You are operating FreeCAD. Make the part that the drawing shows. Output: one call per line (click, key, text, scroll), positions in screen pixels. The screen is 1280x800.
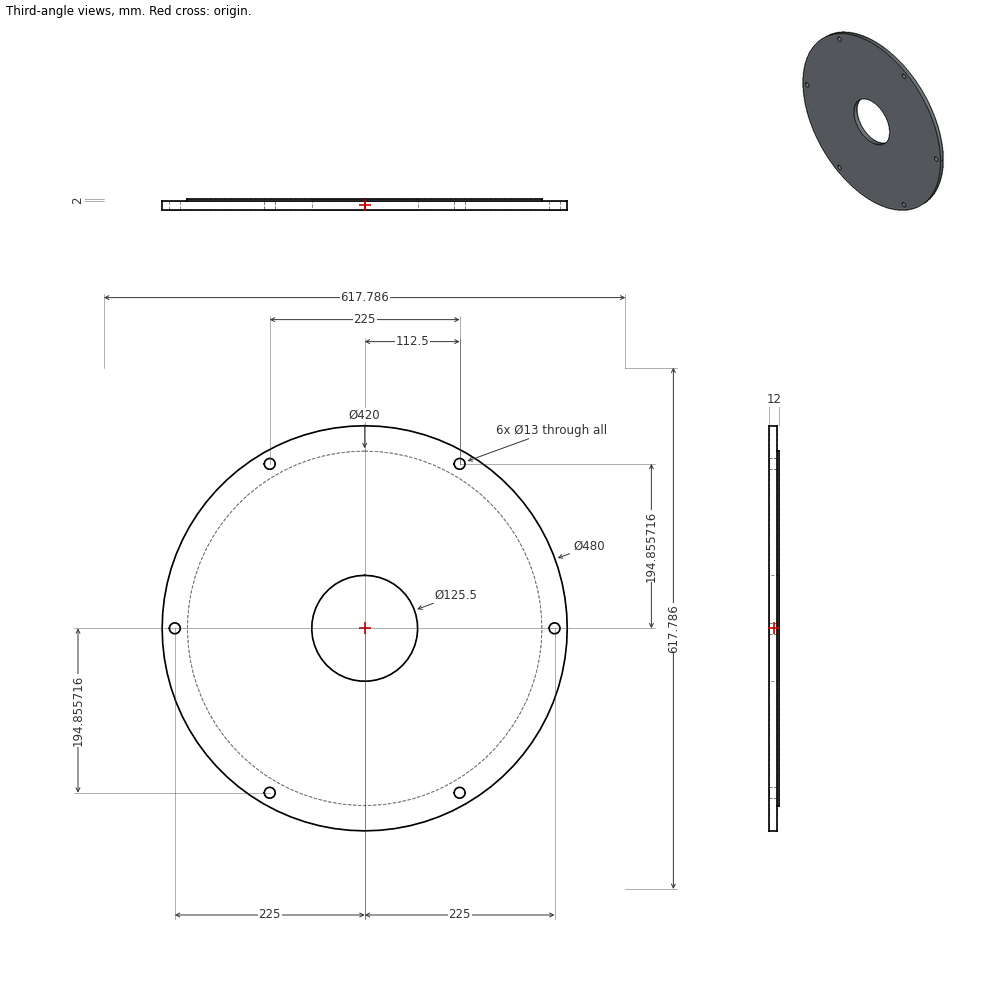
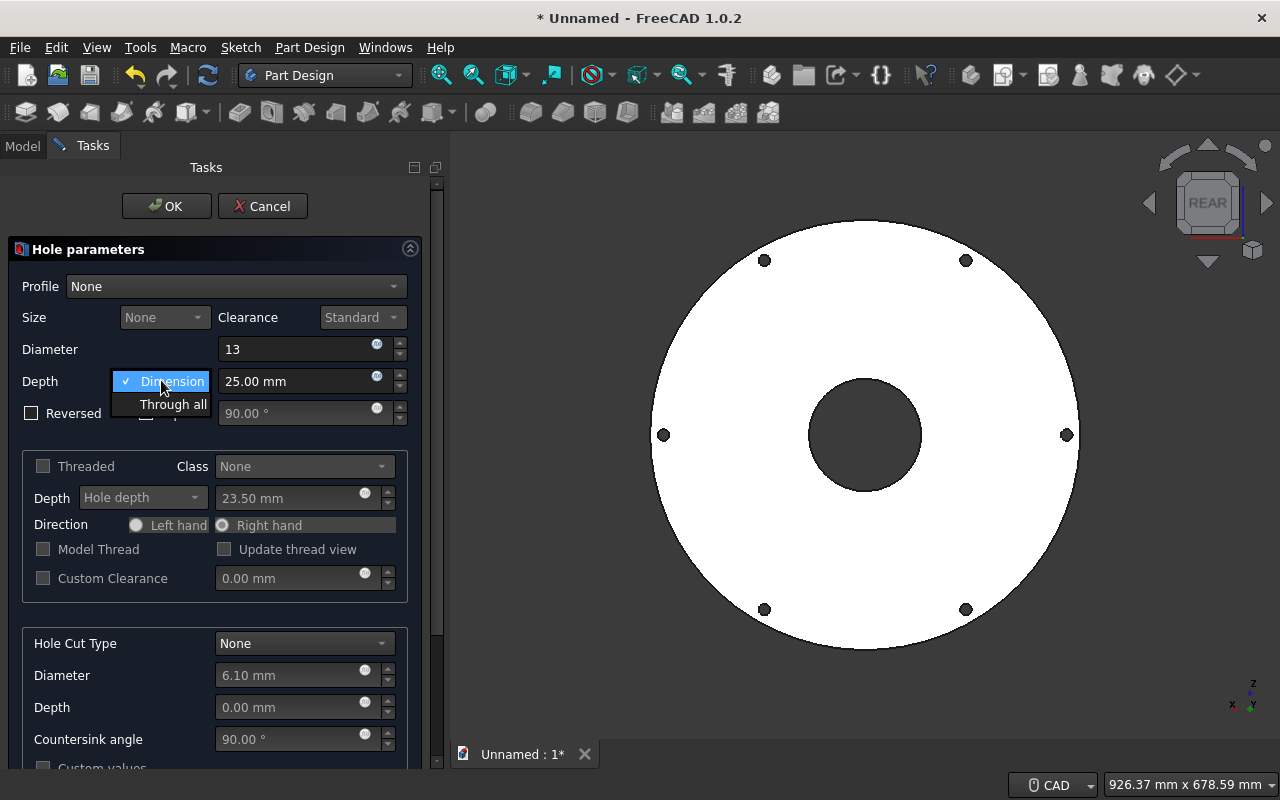
click(160, 404)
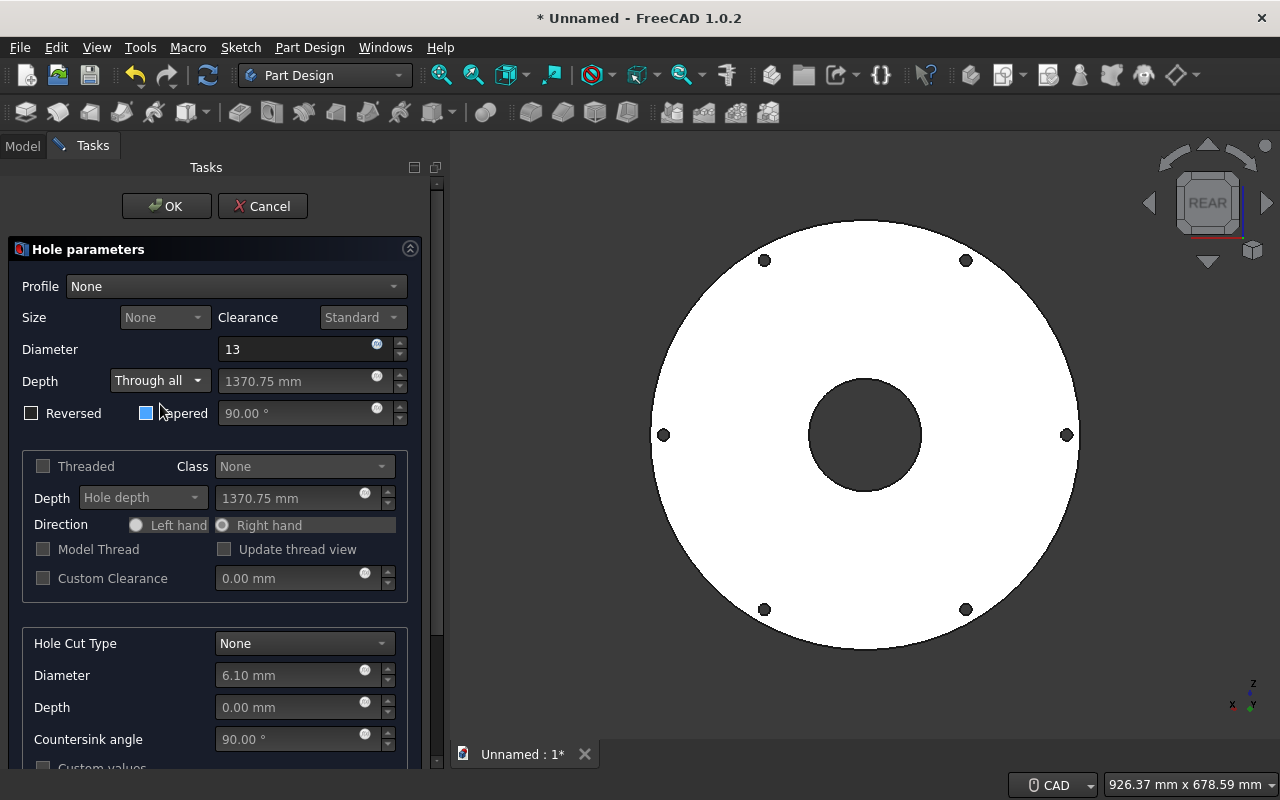
click(167, 206)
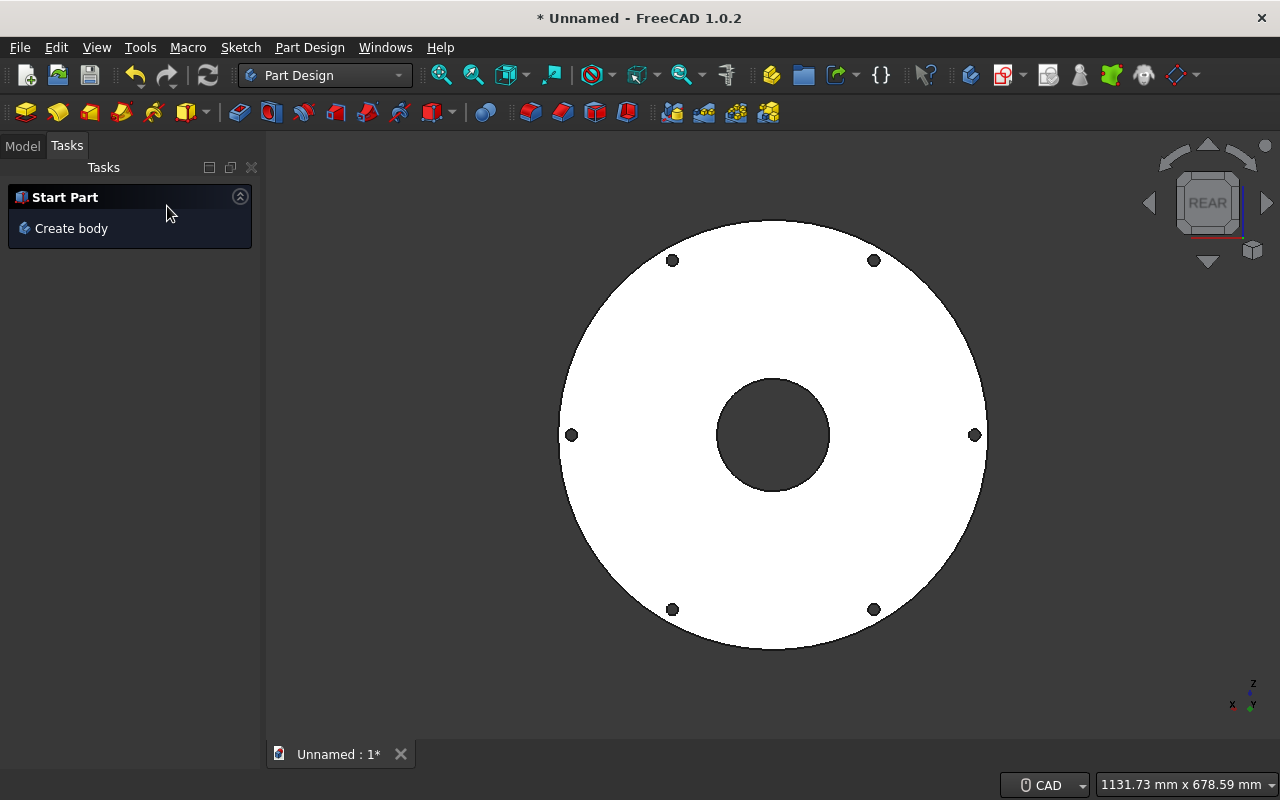
click(896, 373)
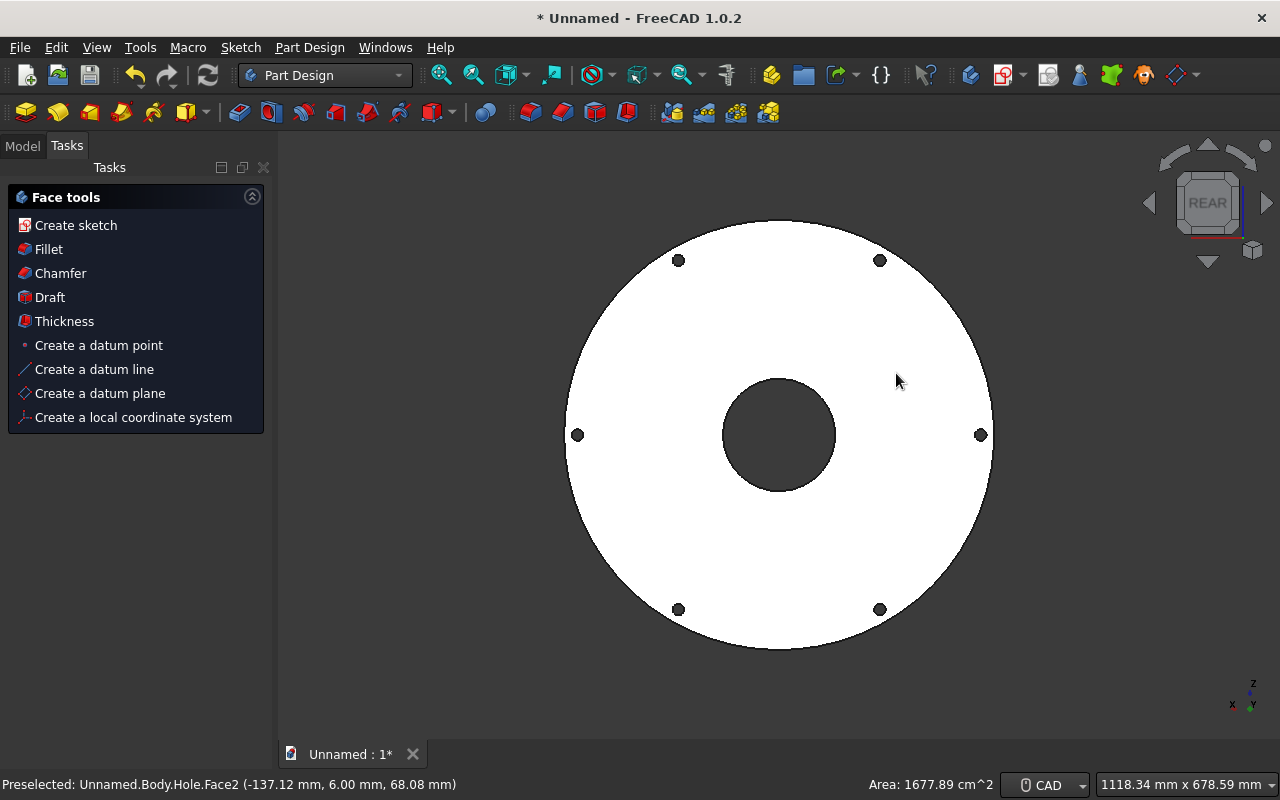
click(1004, 76)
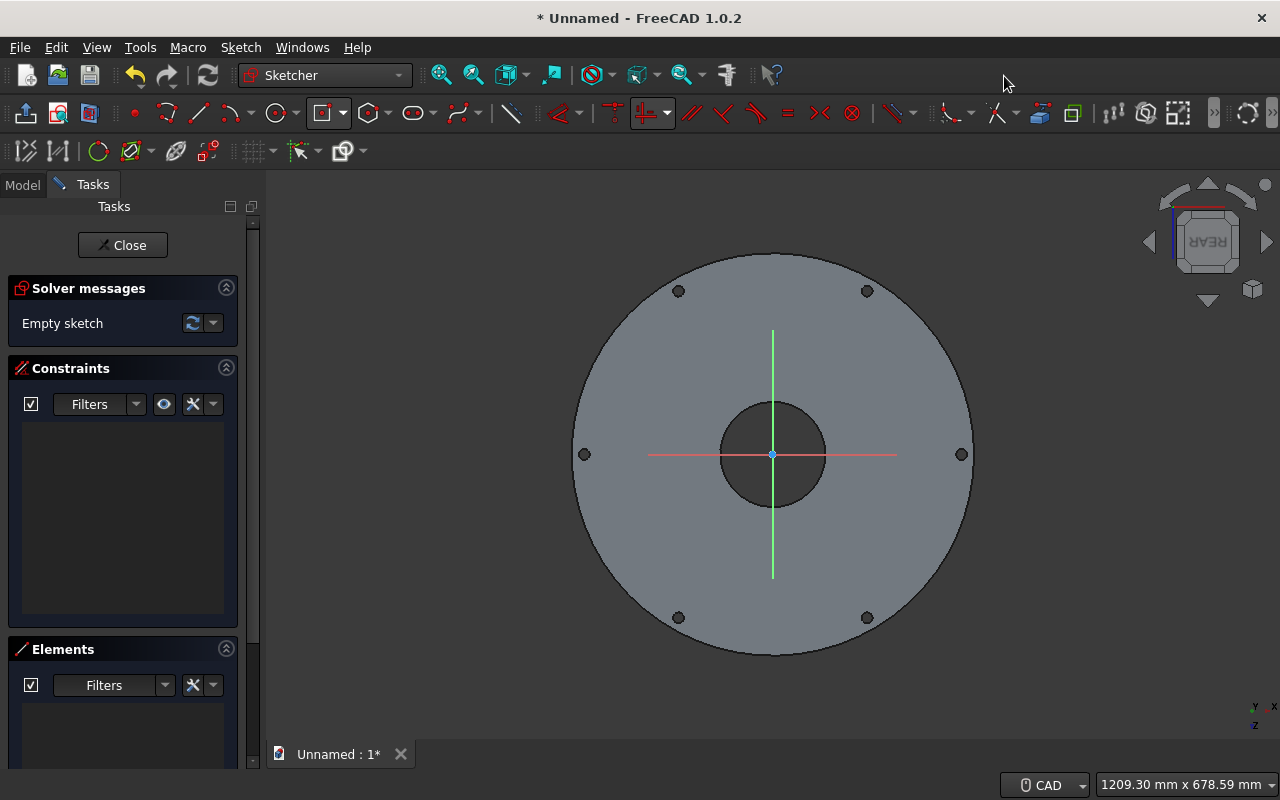
scroll(565, 455, down, 2)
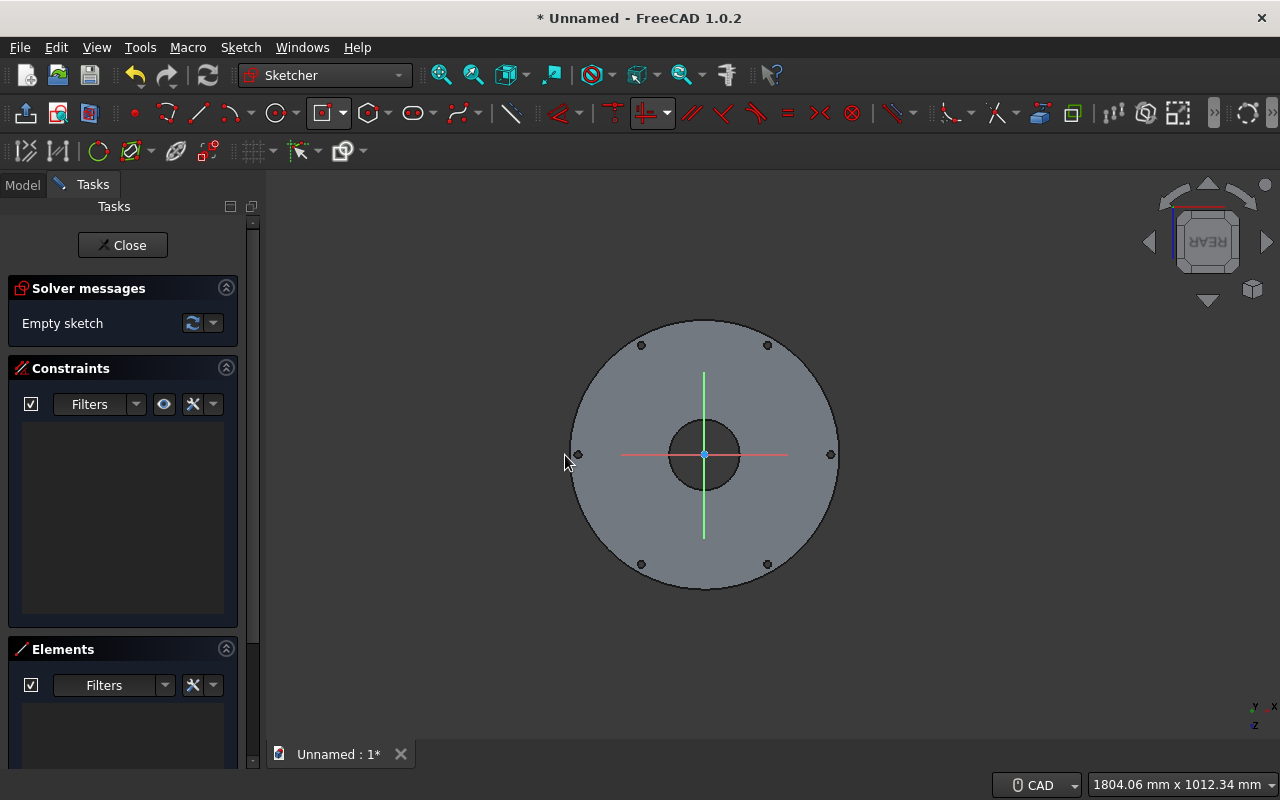
click(322, 114)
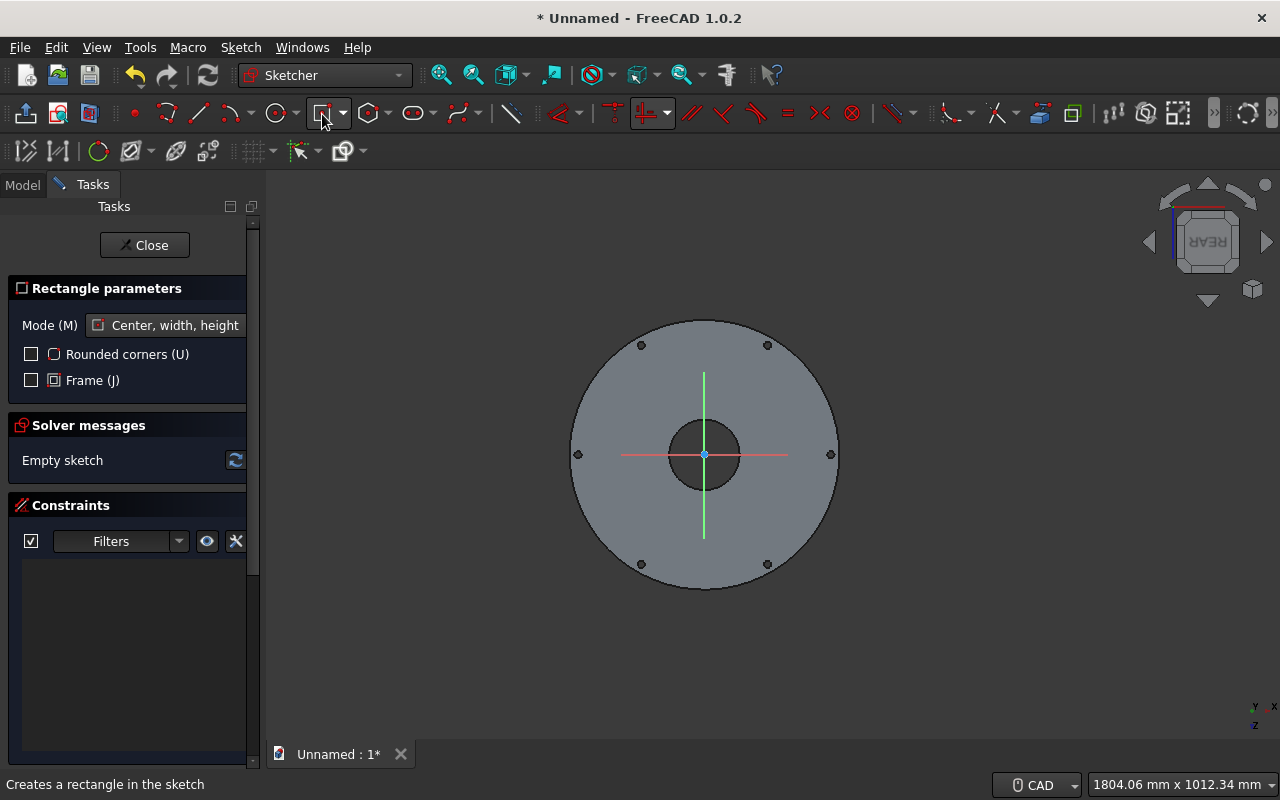
click(704, 455)
move(878, 281)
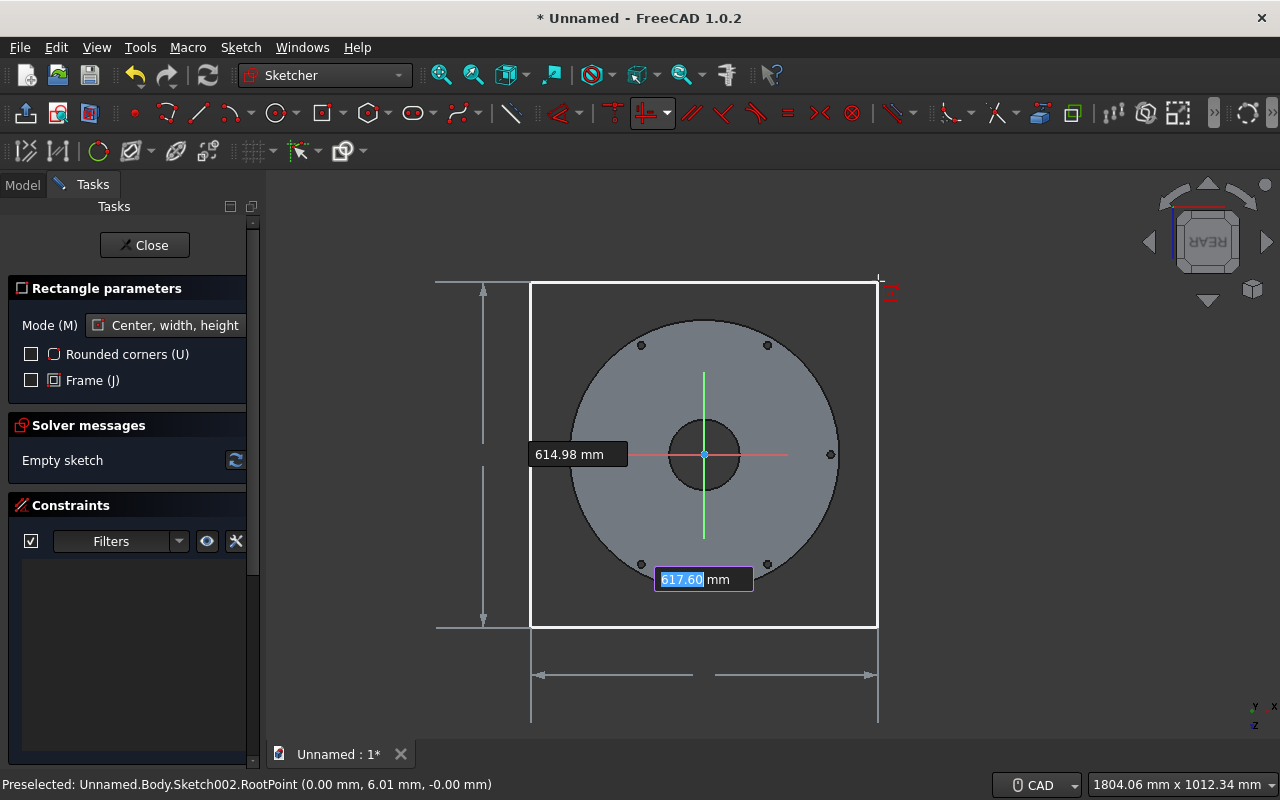
text(617.786)
key(Tab)
text(617.786)
key(Return)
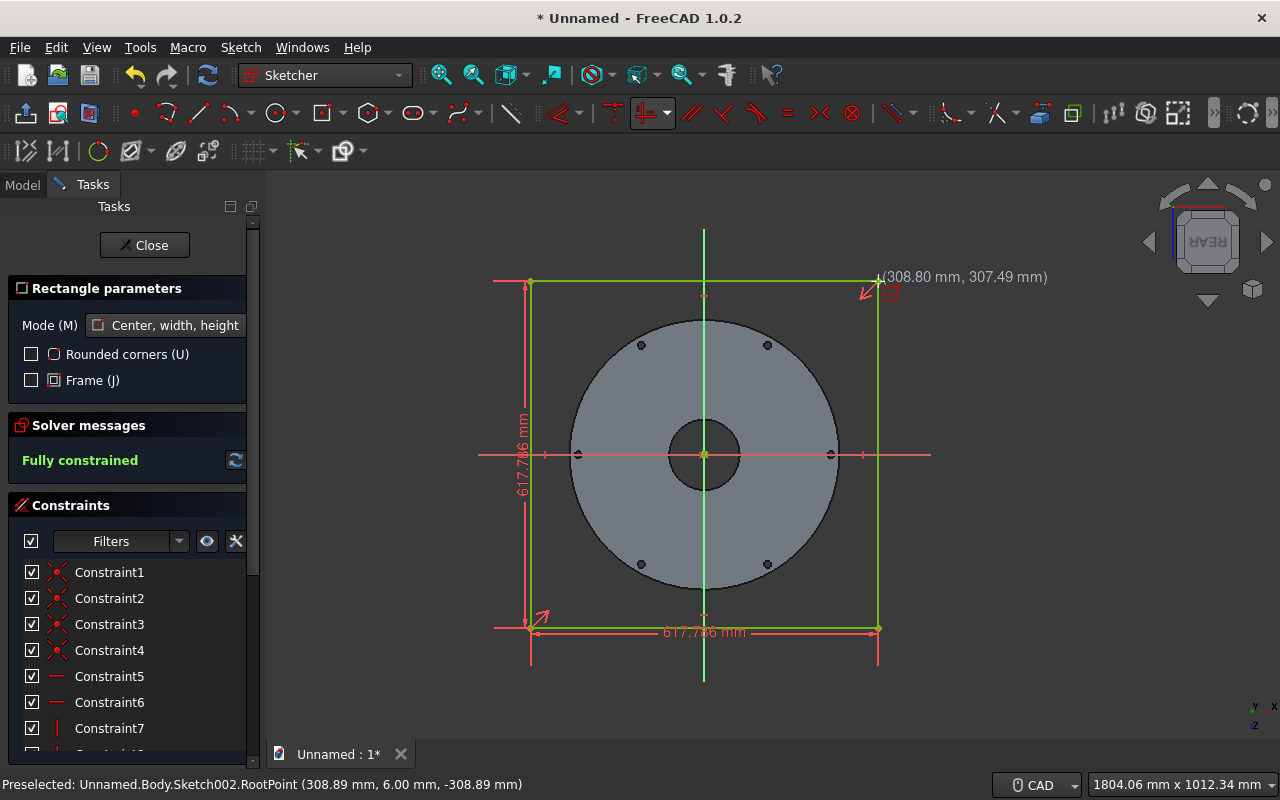
click(276, 114)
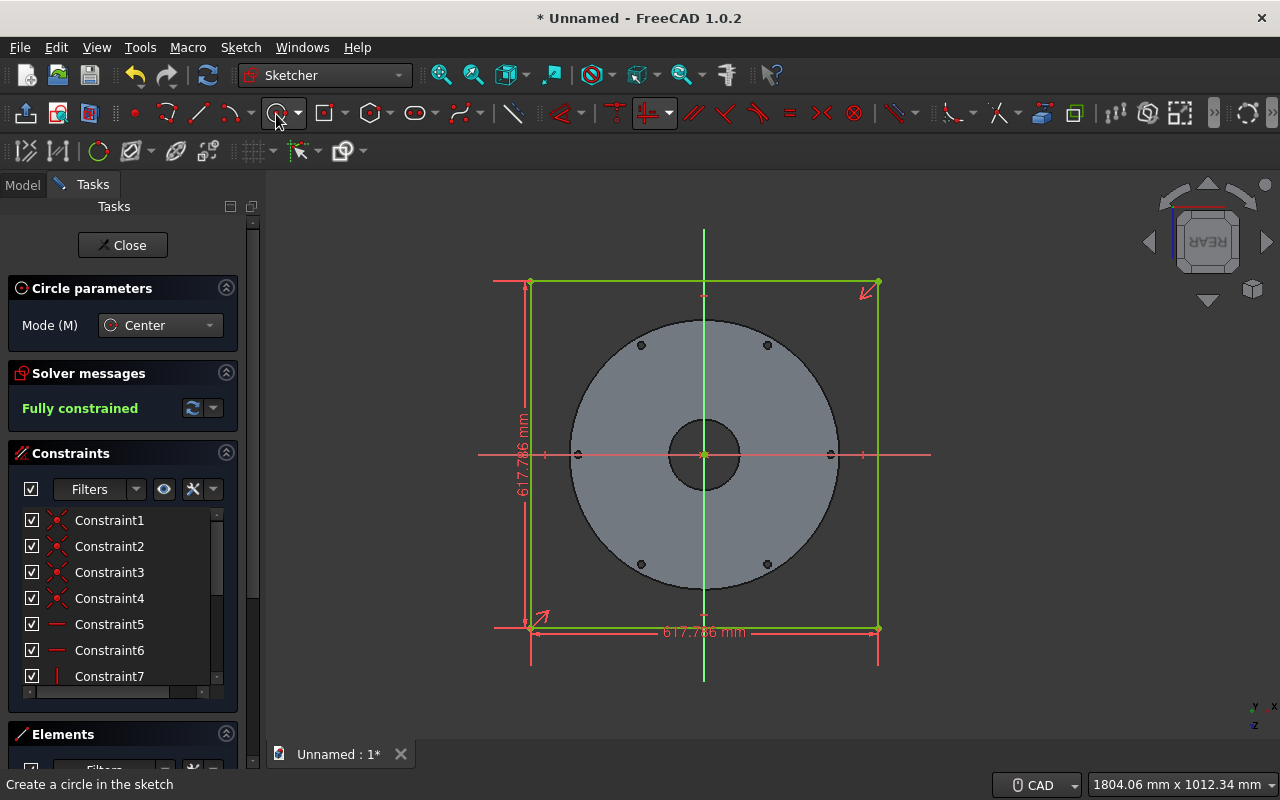
click(704, 455)
move(788, 371)